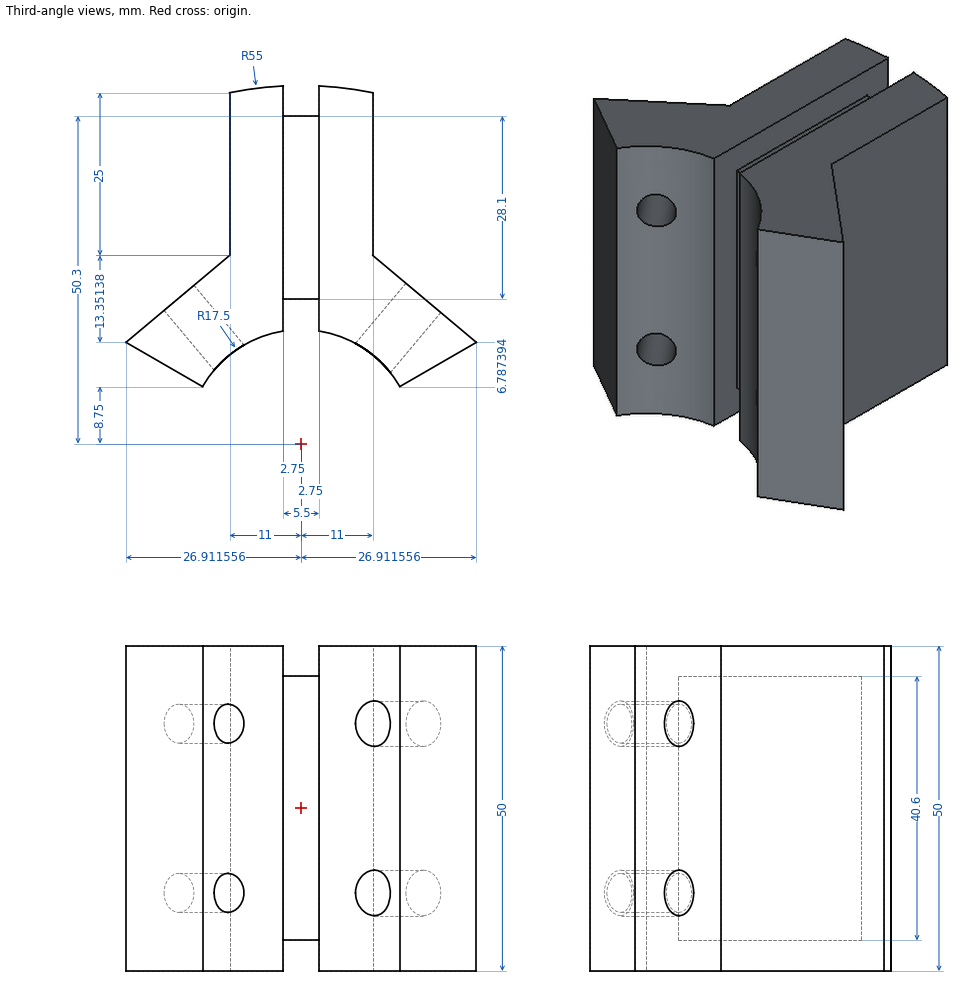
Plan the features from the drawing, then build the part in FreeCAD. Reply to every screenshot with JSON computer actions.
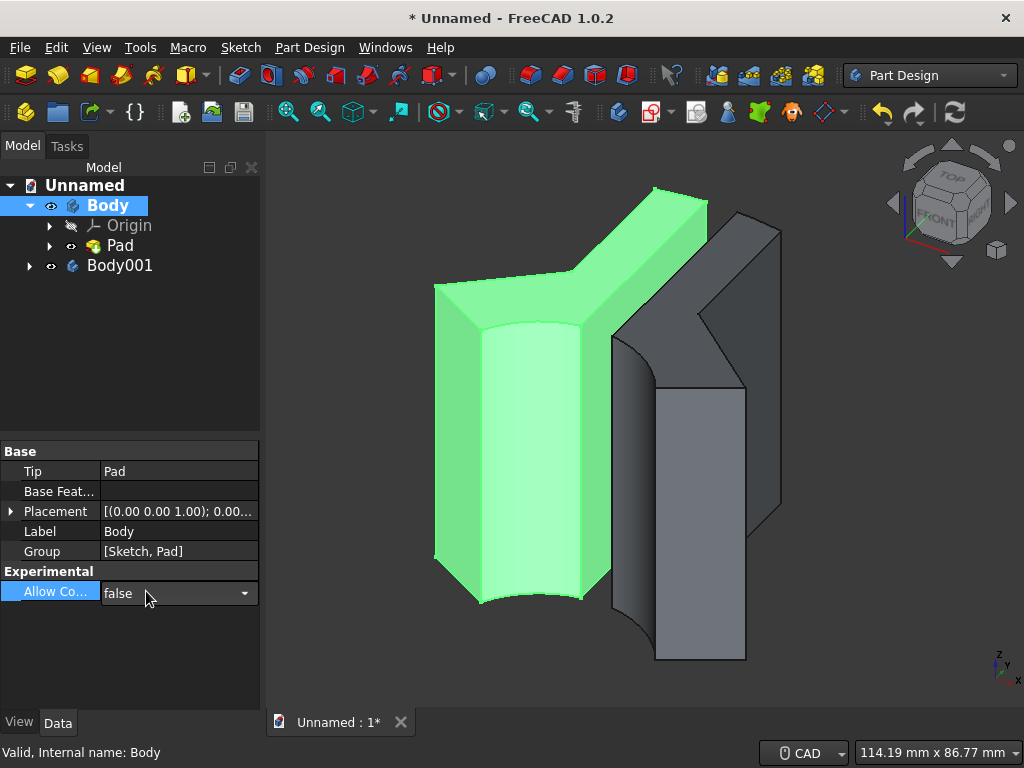
{"action": "left_click", "coordinate": [146, 591]}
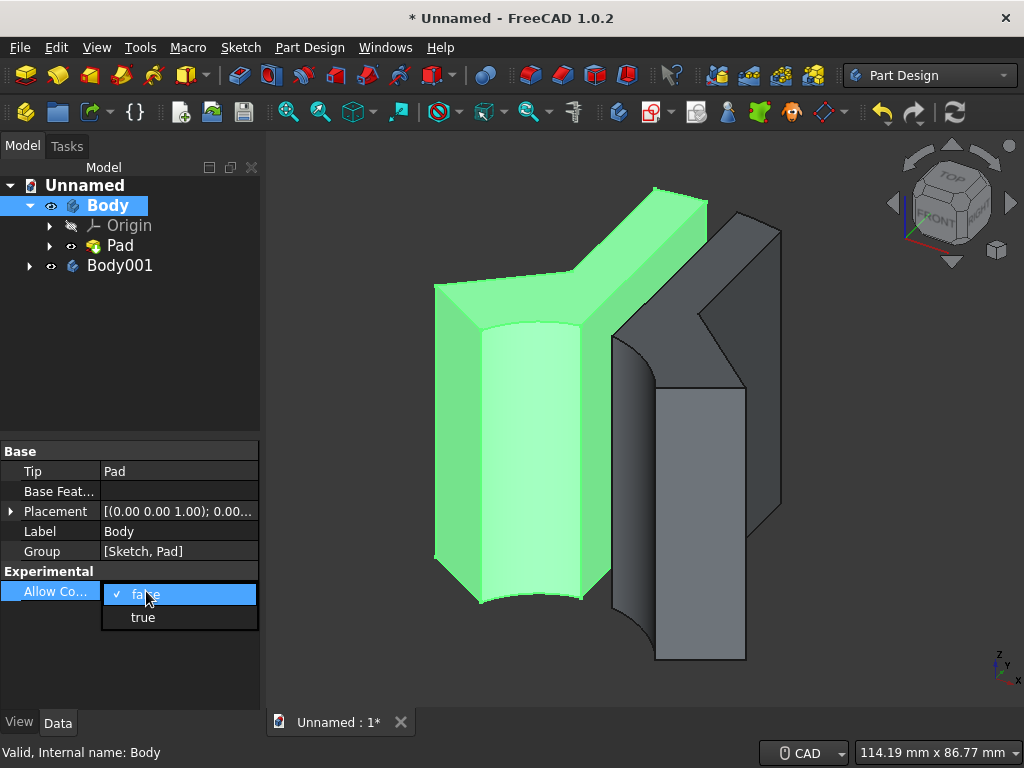
{"action": "left_click", "coordinate": [179, 618]}
{"action": "key", "text": "Return"}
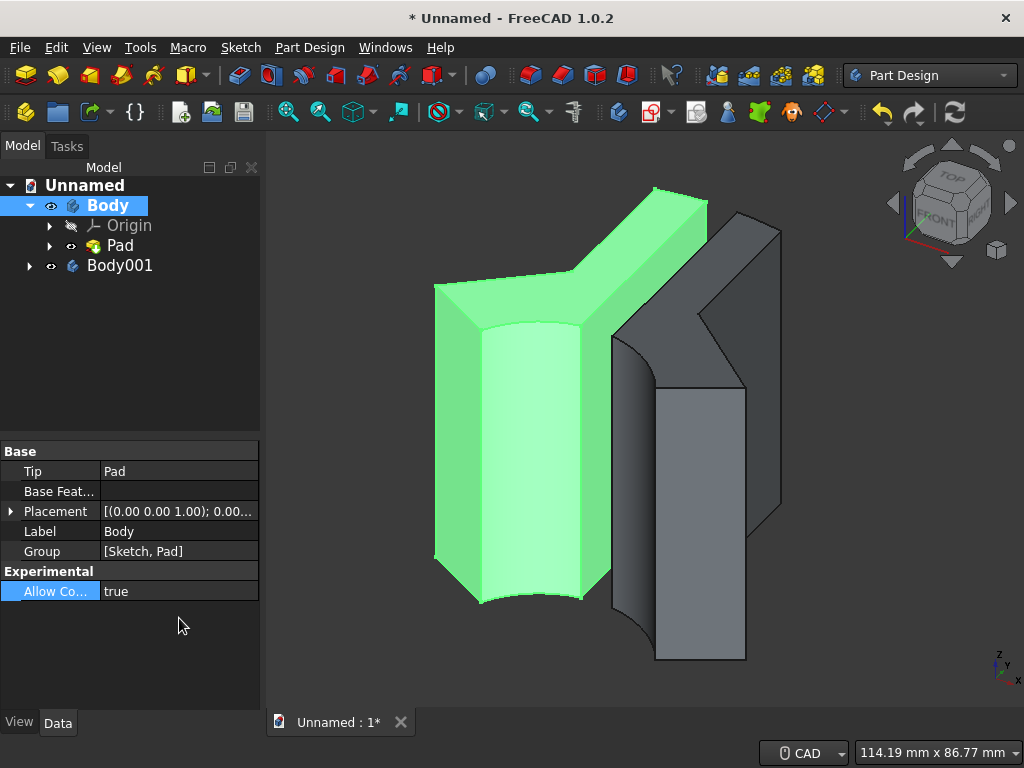
{"action": "left_click", "coordinate": [96, 266]}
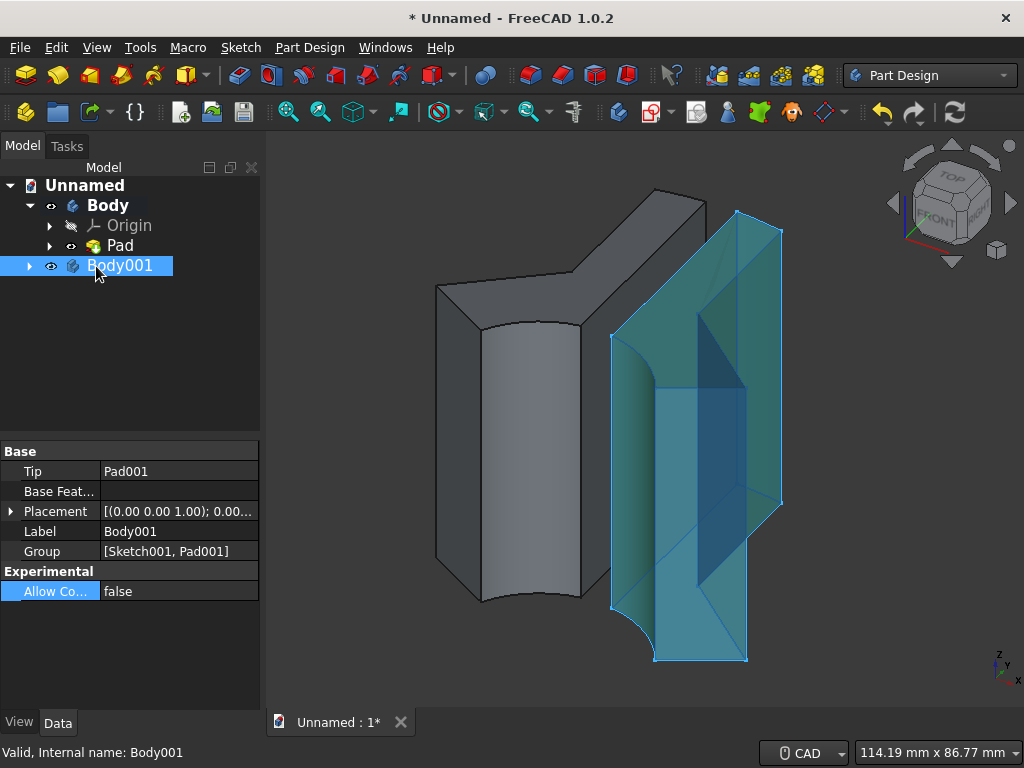
{"action": "left_click", "coordinate": [486, 76]}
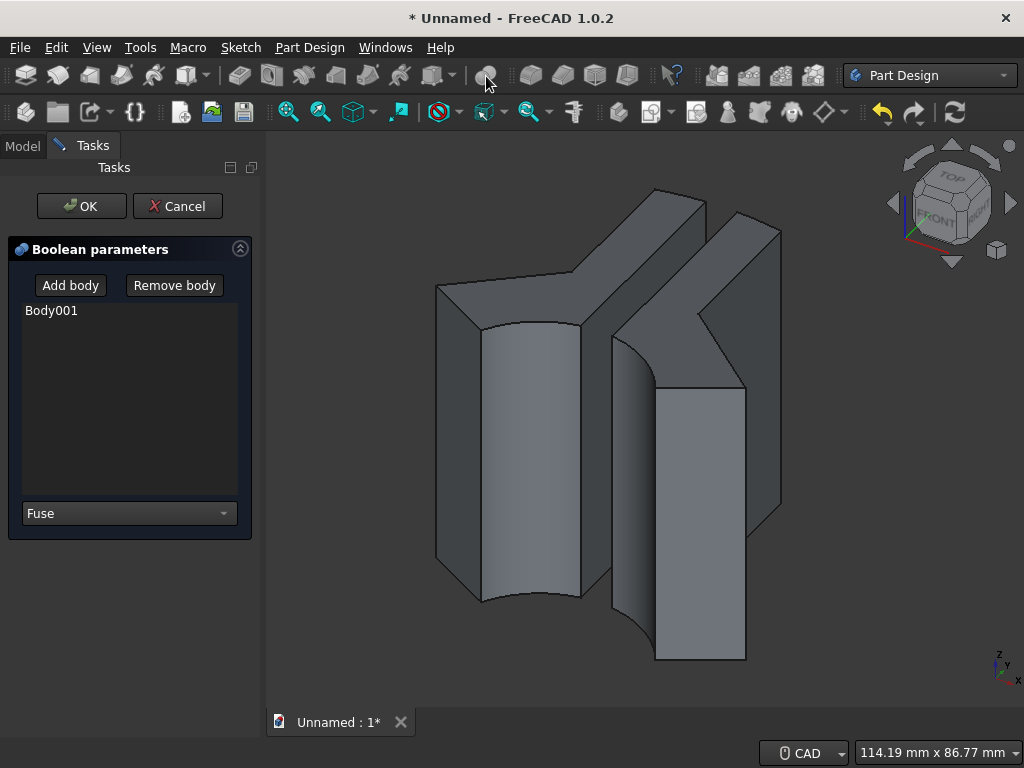
{"action": "left_click", "coordinate": [82, 206]}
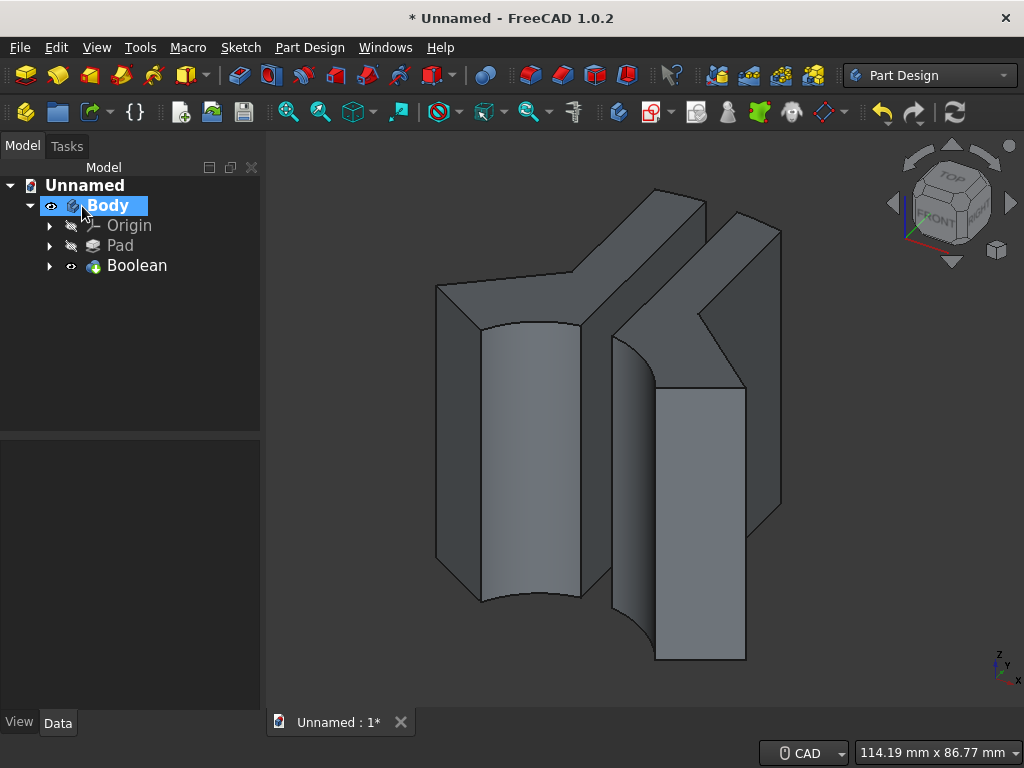
{"action": "left_click", "coordinate": [652, 112]}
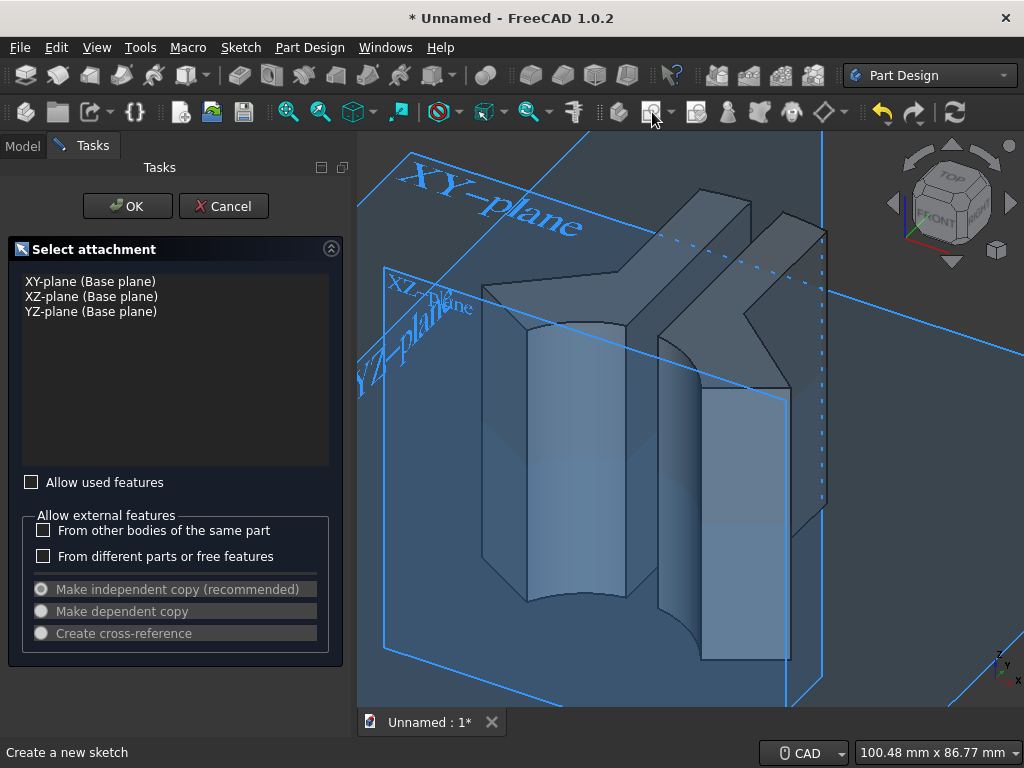
{"action": "left_click", "coordinate": [82, 282]}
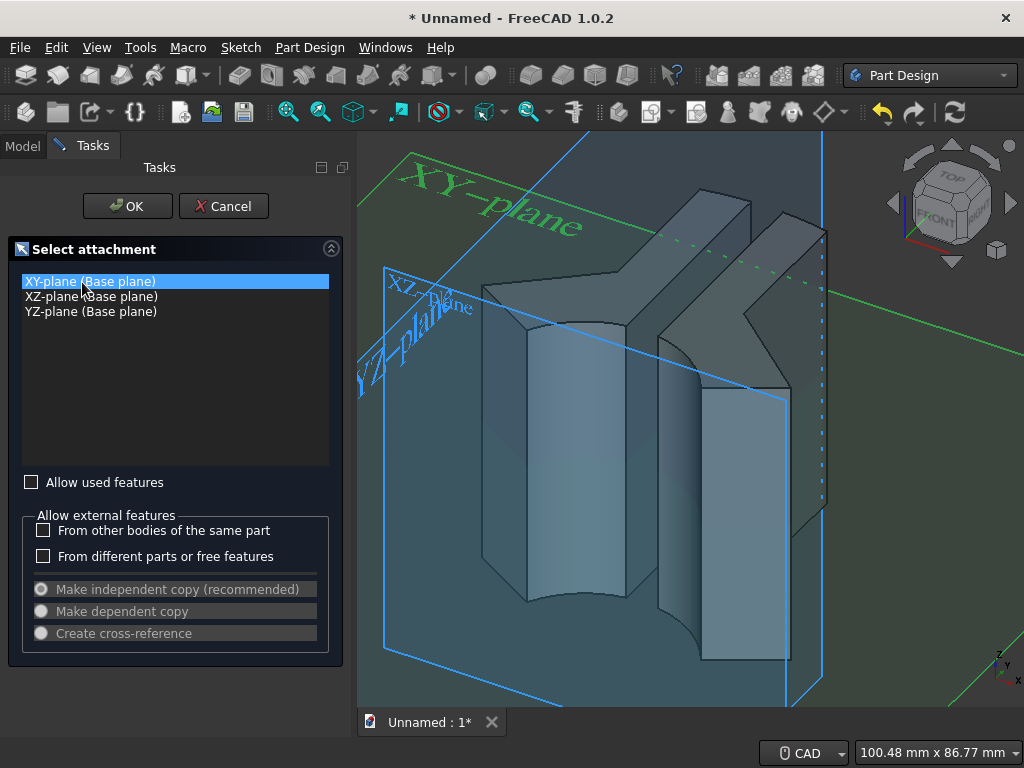
{"action": "left_click", "coordinate": [128, 206]}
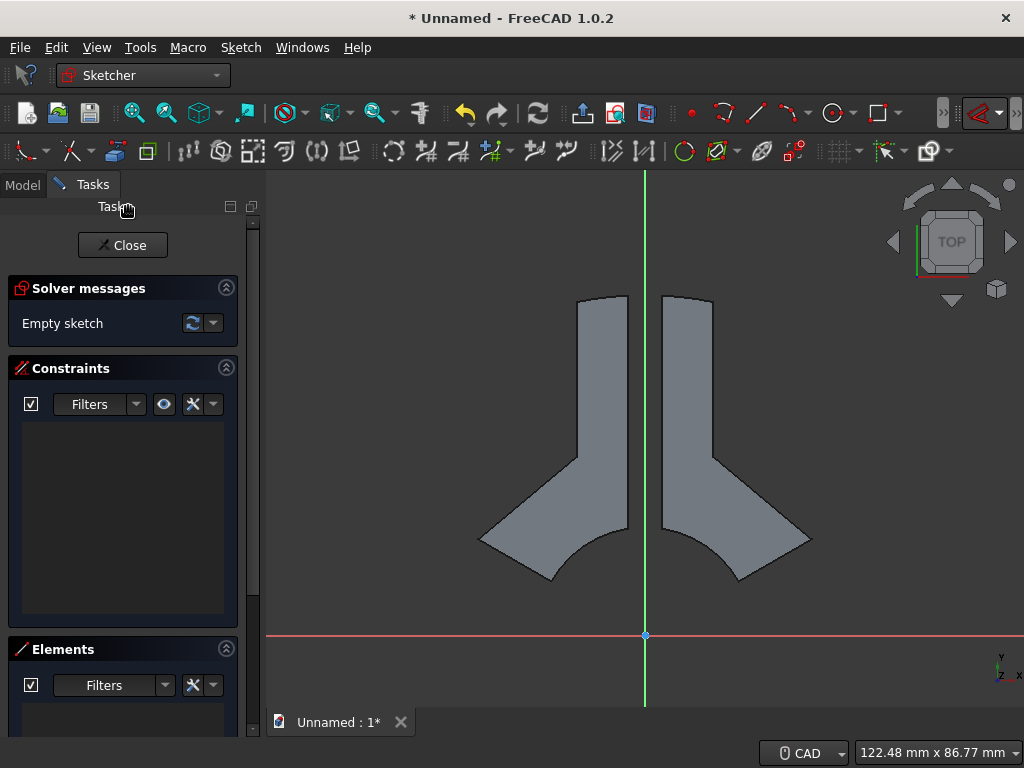
{"action": "left_click", "coordinate": [648, 114]}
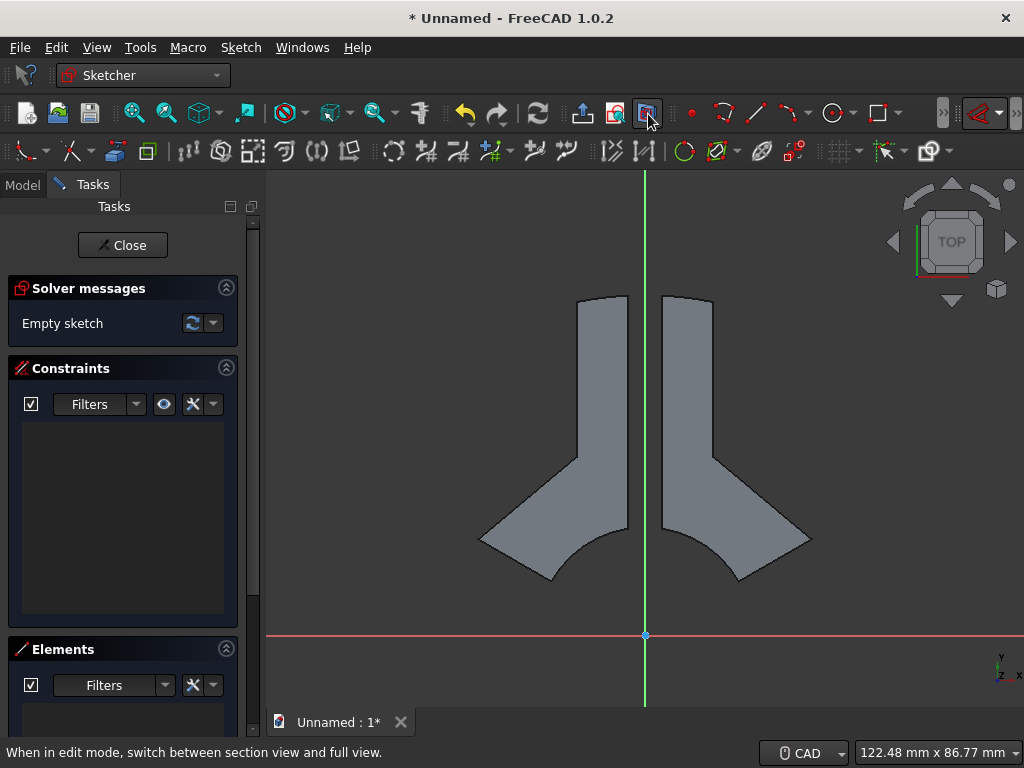
{"action": "left_click", "coordinate": [878, 114]}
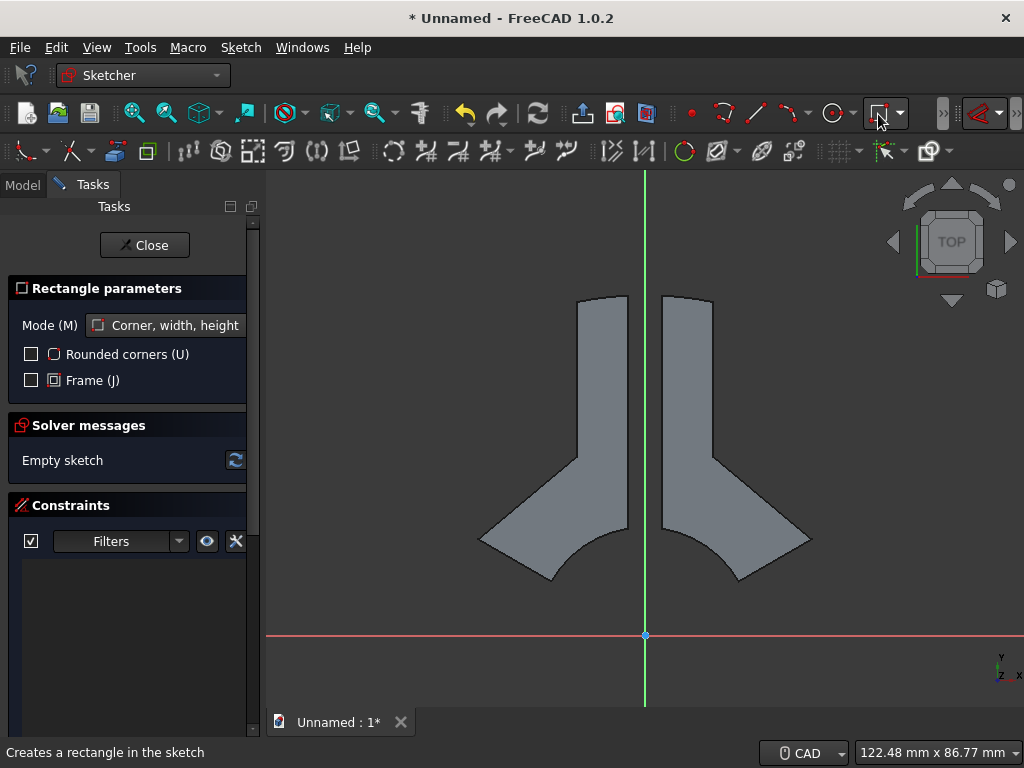
{"action": "left_click", "coordinate": [628, 324]}
{"action": "mouse_move", "coordinate": [662, 498]}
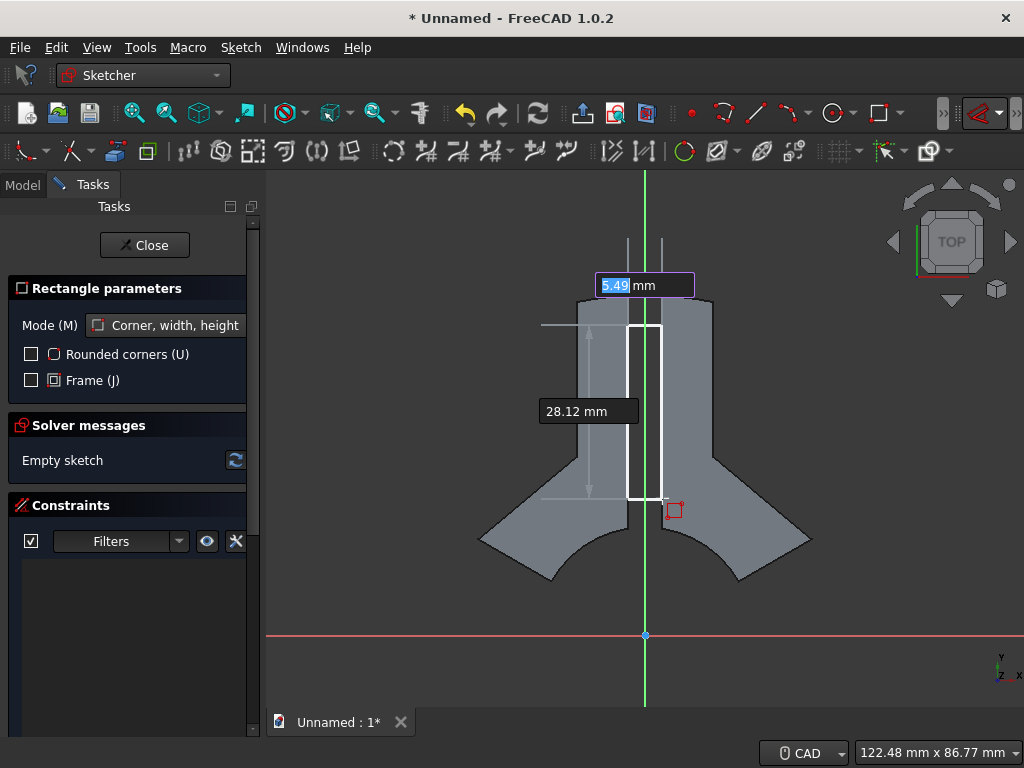
{"action": "type", "text": "5.5"}
{"action": "key", "text": "Tab"}
{"action": "type", "text": "28.1"}
{"action": "key", "text": "Return"}
{"action": "key", "text": "Escape"}